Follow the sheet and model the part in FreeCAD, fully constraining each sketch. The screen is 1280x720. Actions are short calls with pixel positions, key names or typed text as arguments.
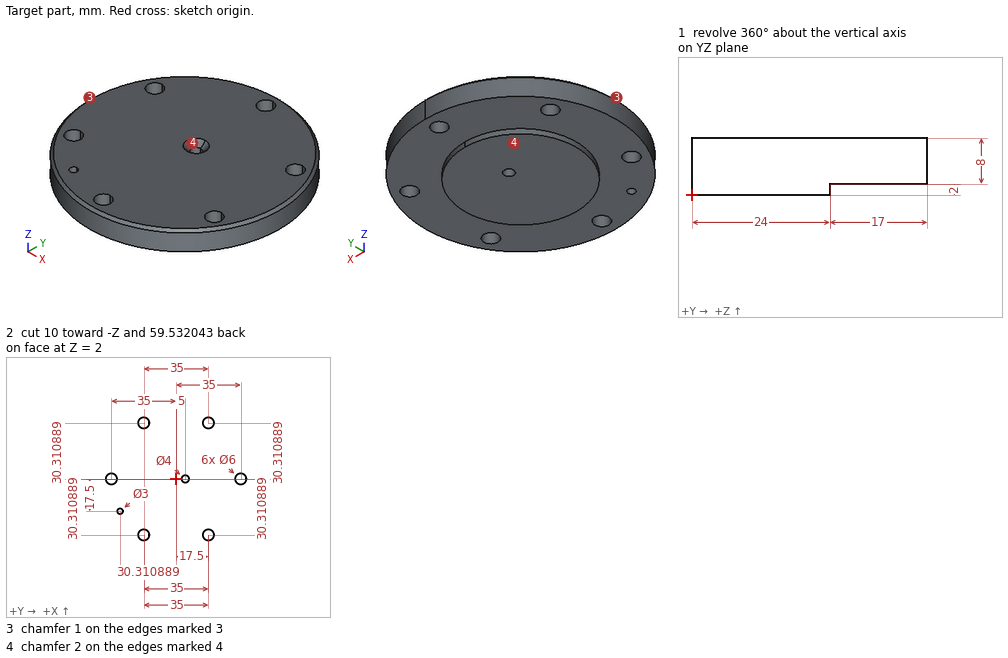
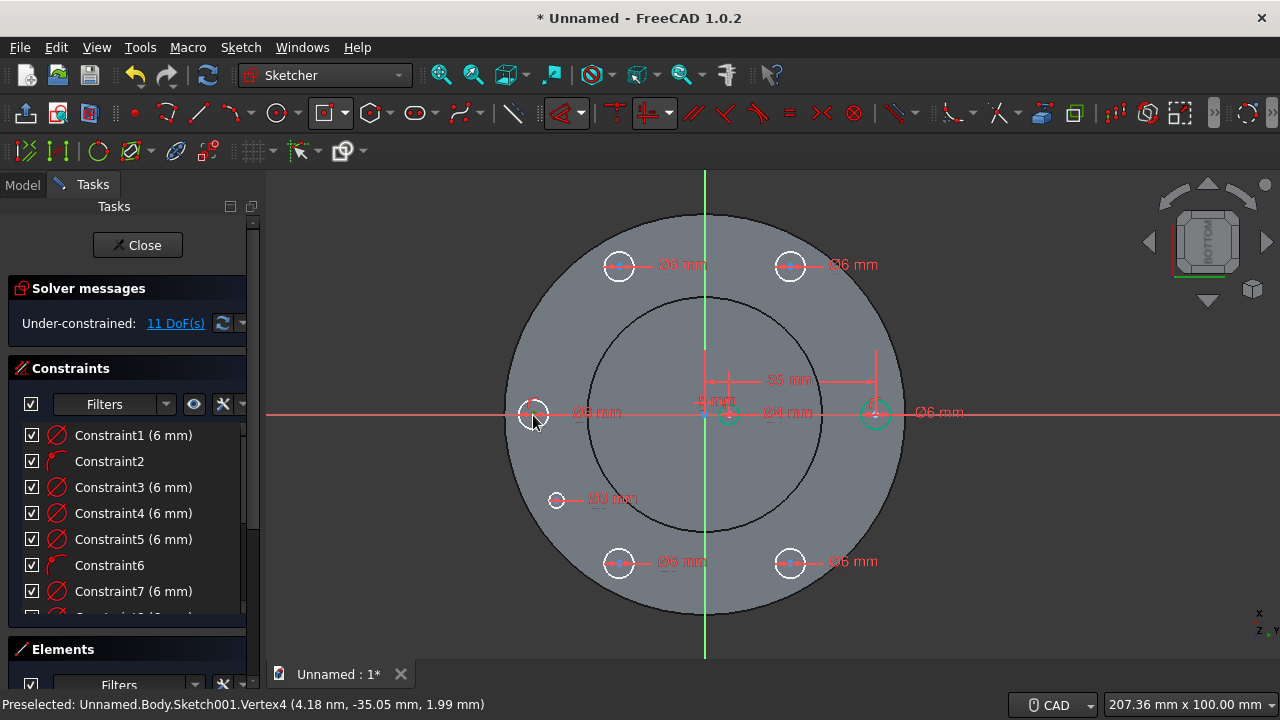
key(l)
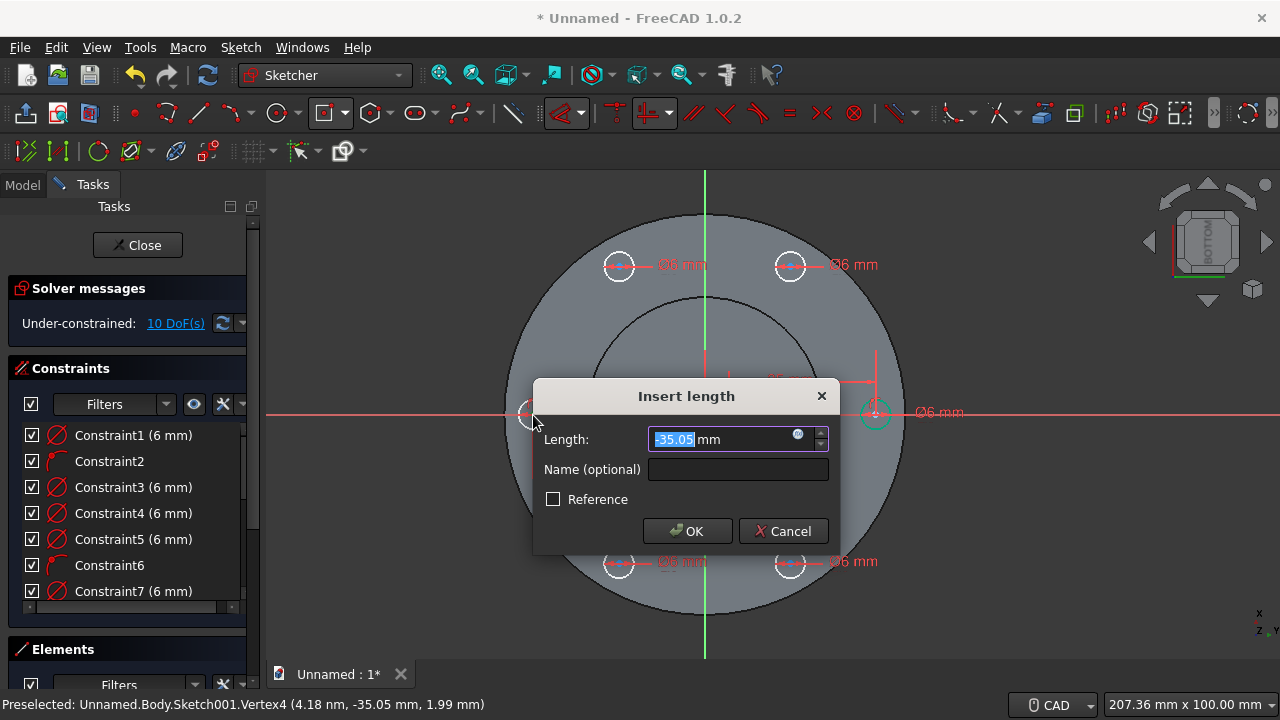
text(-35)
key(Return)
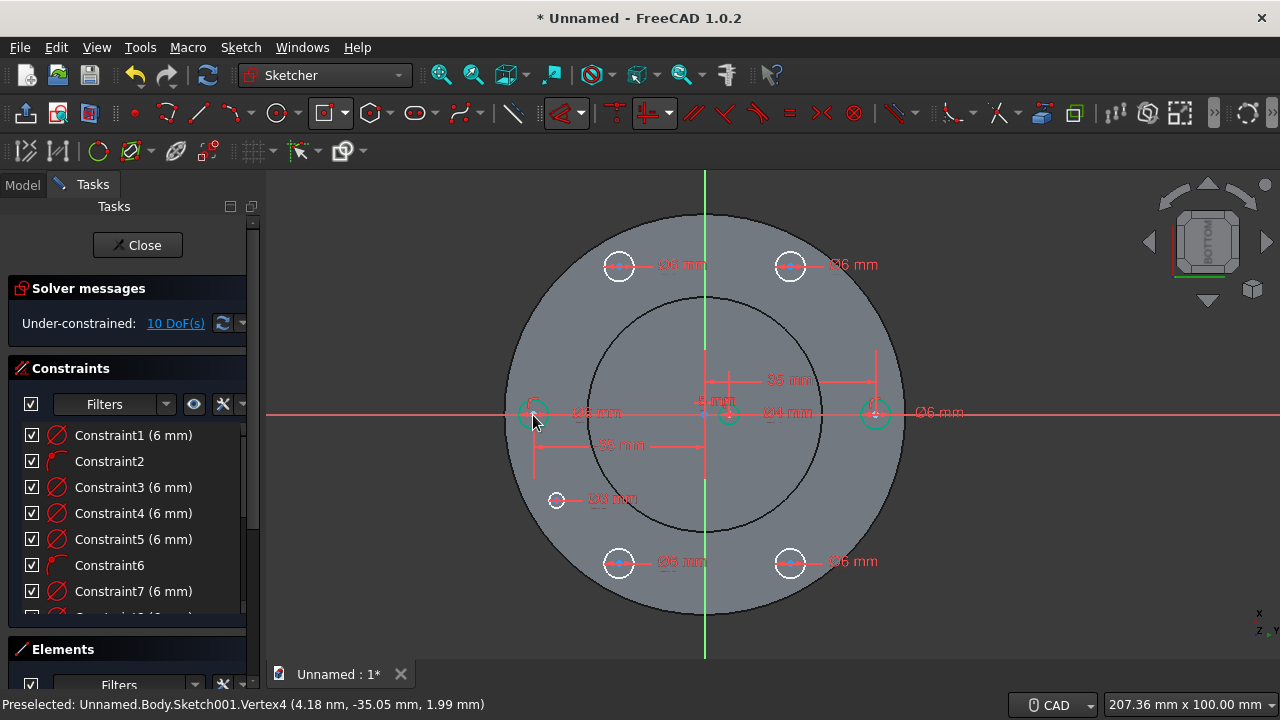
click(790, 564)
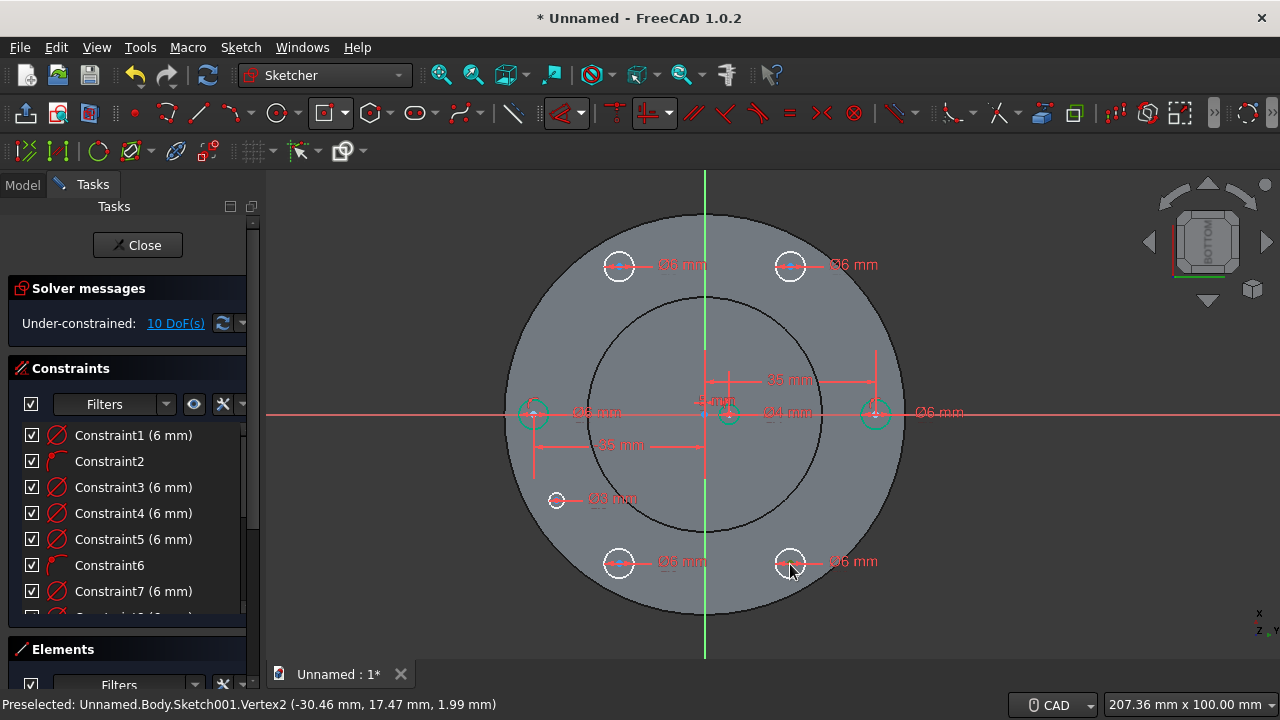
click(619, 564)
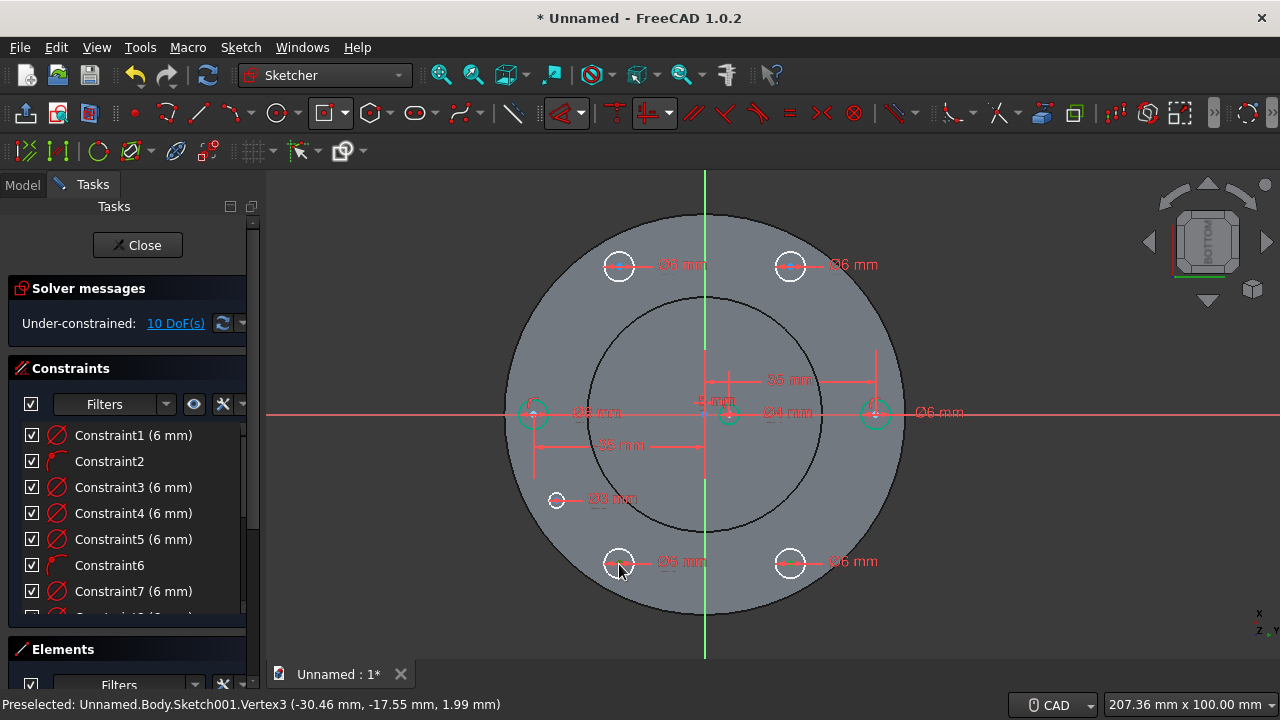
click(584, 114)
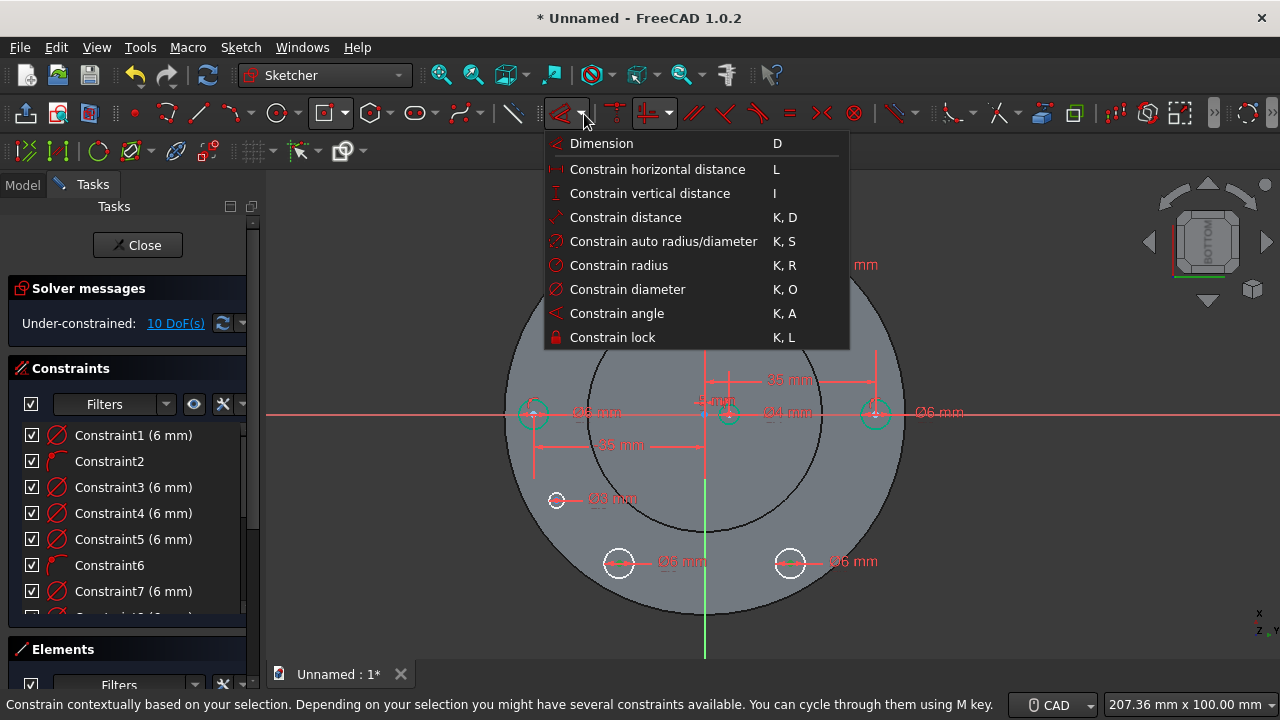
click(697, 169)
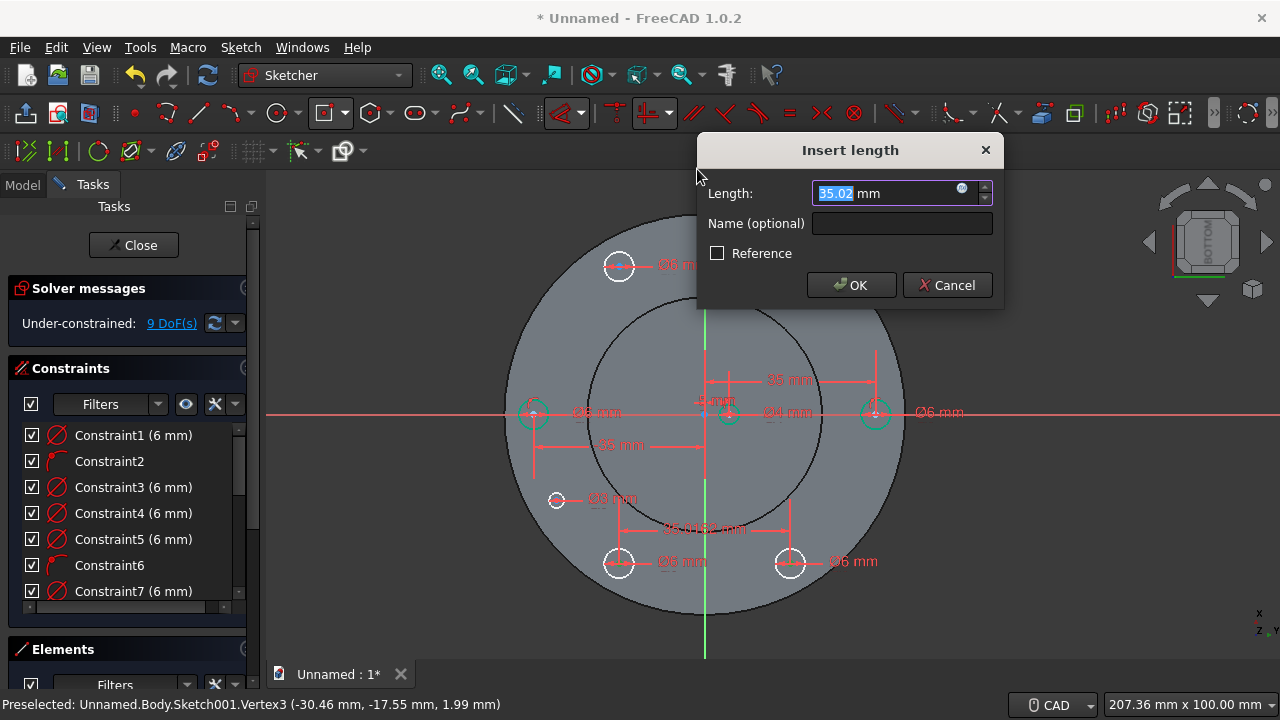
text(35)
key(Return)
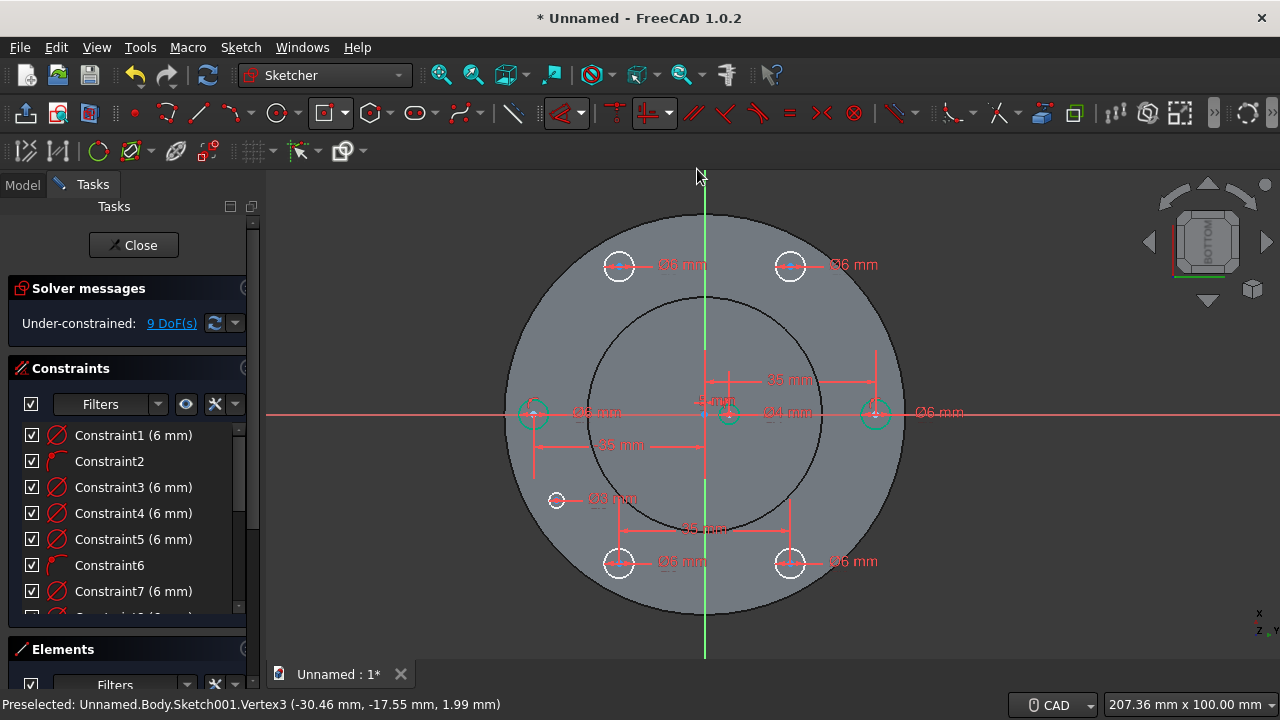
click(790, 564)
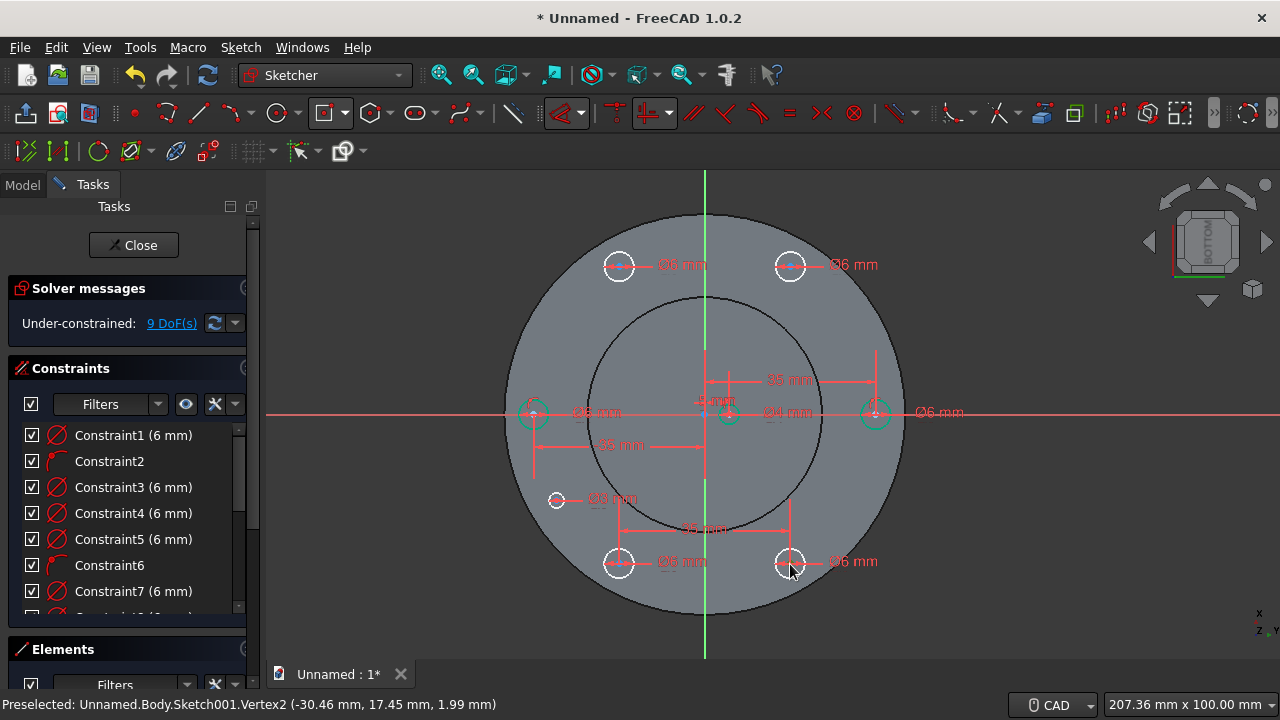
click(619, 267)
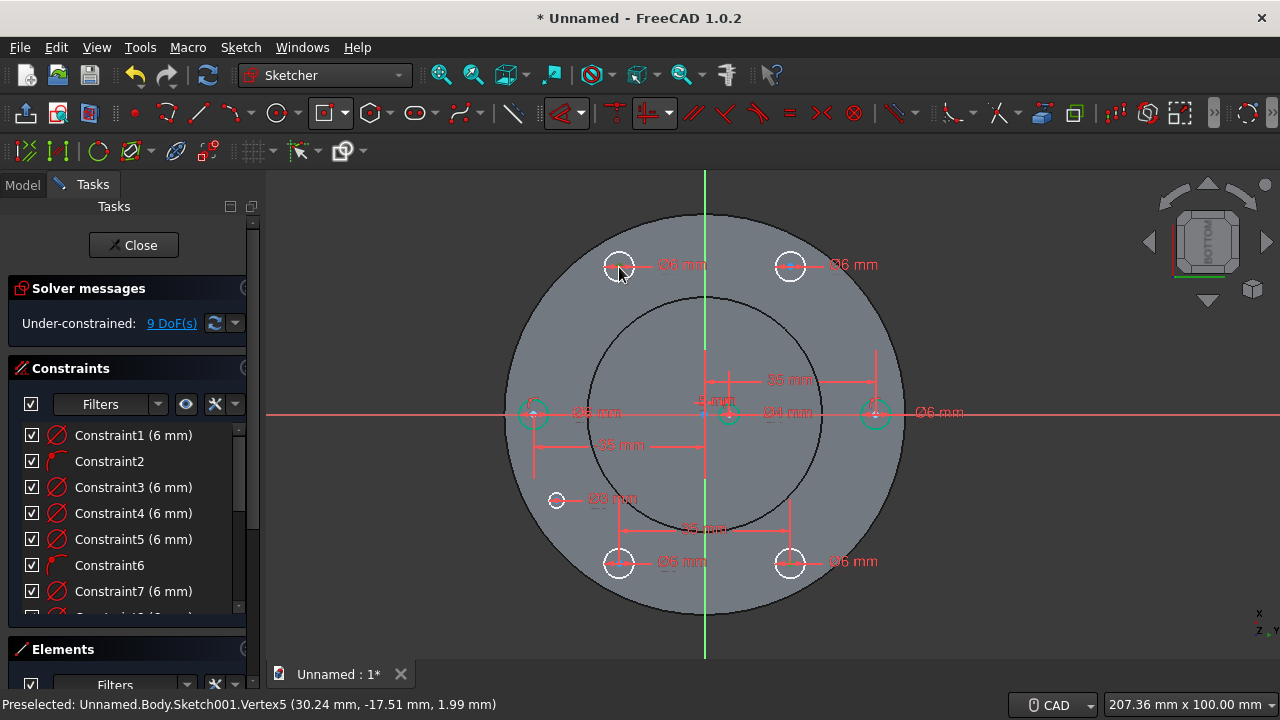
click(584, 114)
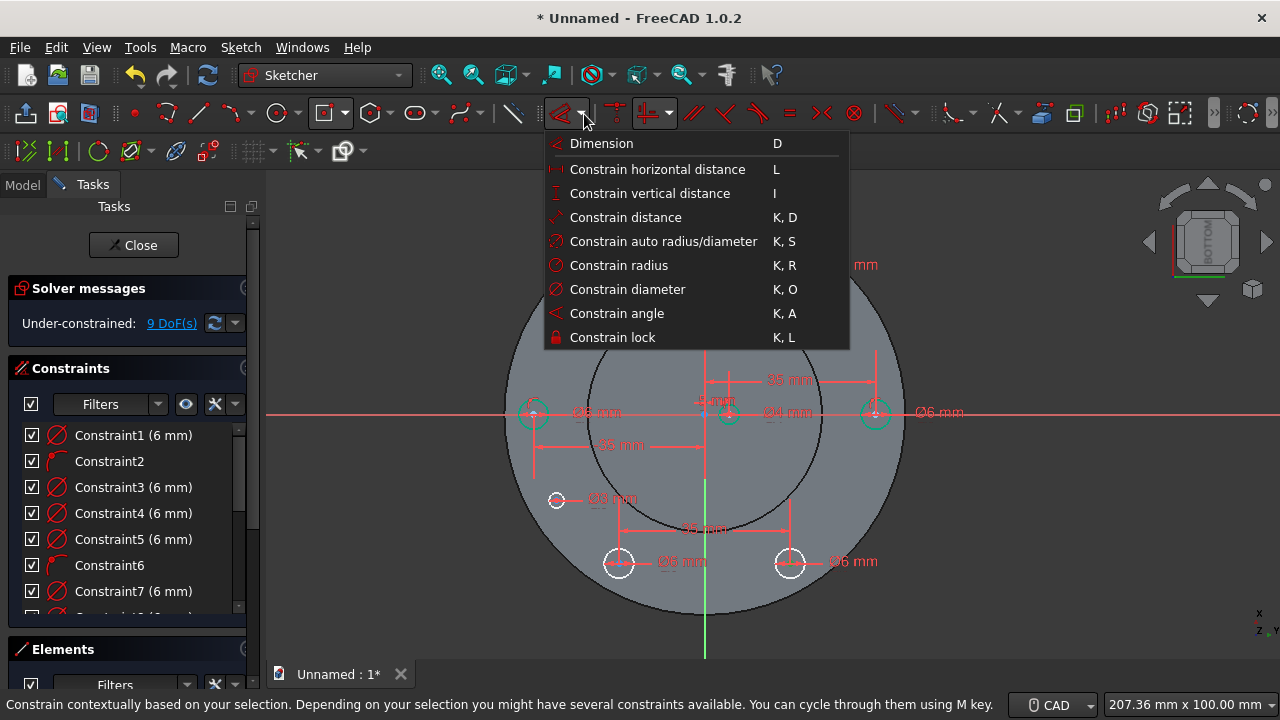
click(697, 169)